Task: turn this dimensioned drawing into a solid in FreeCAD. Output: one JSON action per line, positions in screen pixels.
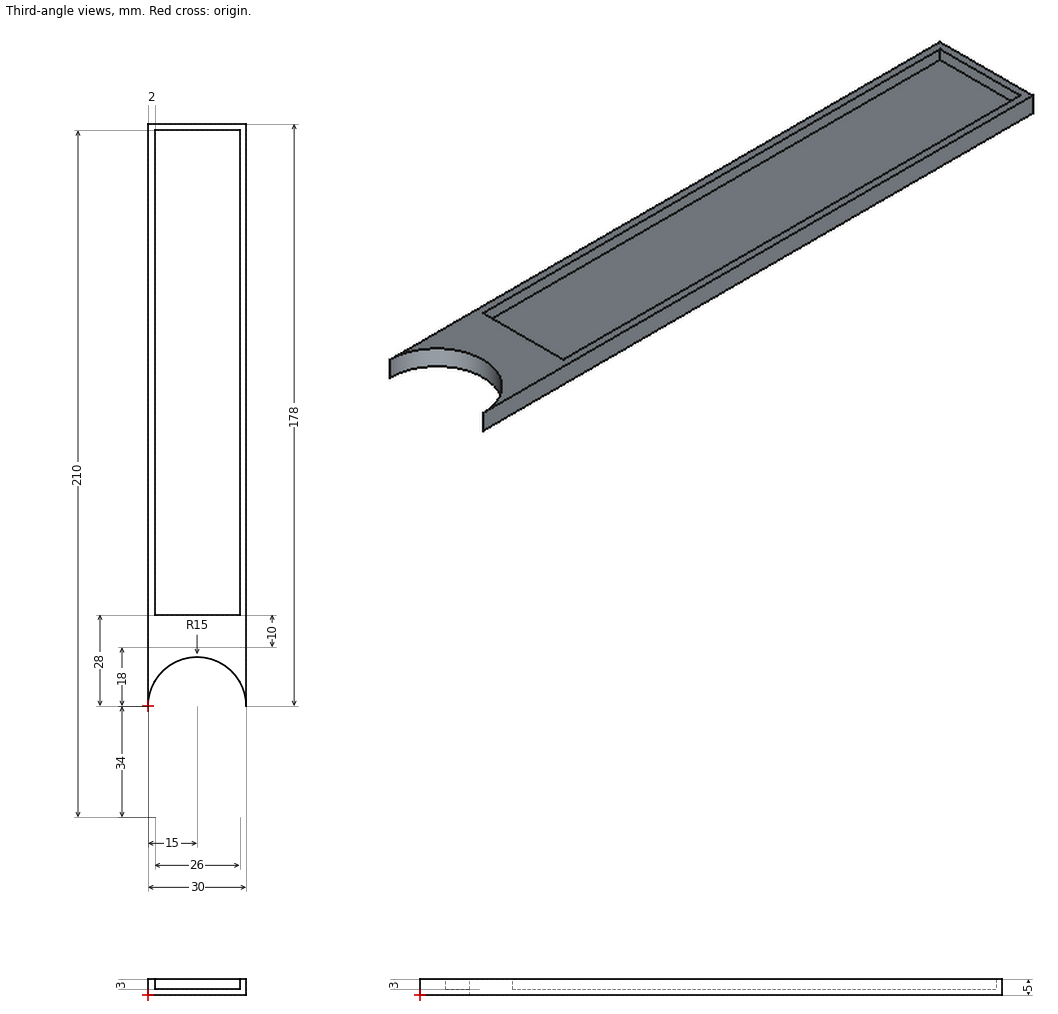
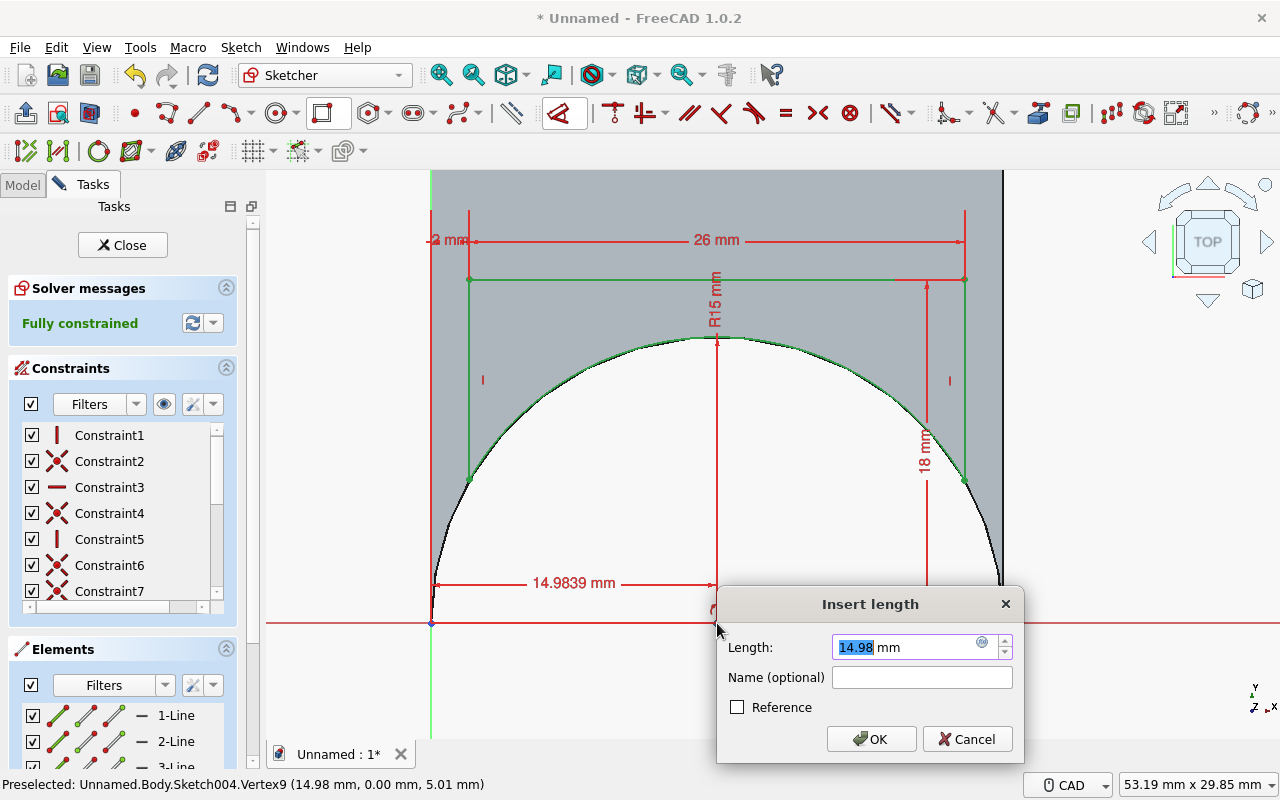
{"action": "type", "text": "15"}
{"action": "key", "text": "Return"}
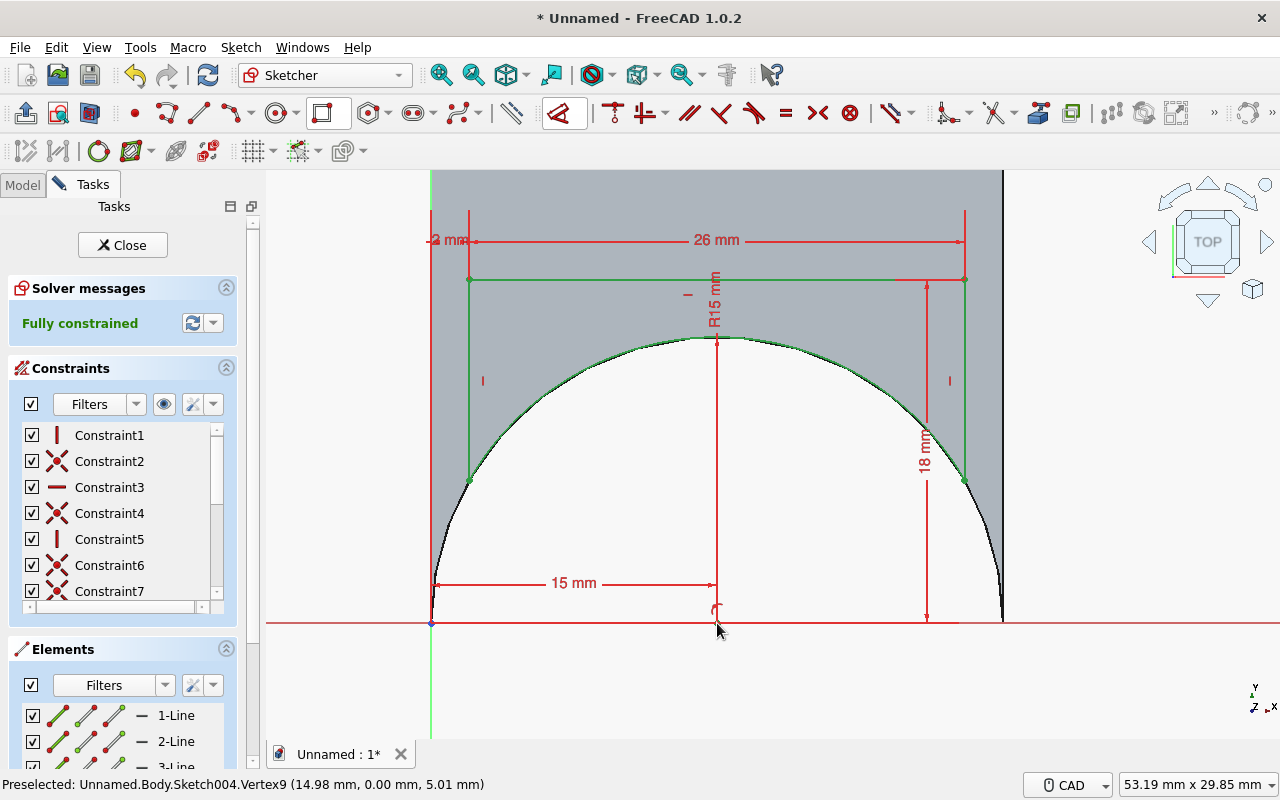
{"action": "left_click", "coordinate": [123, 245]}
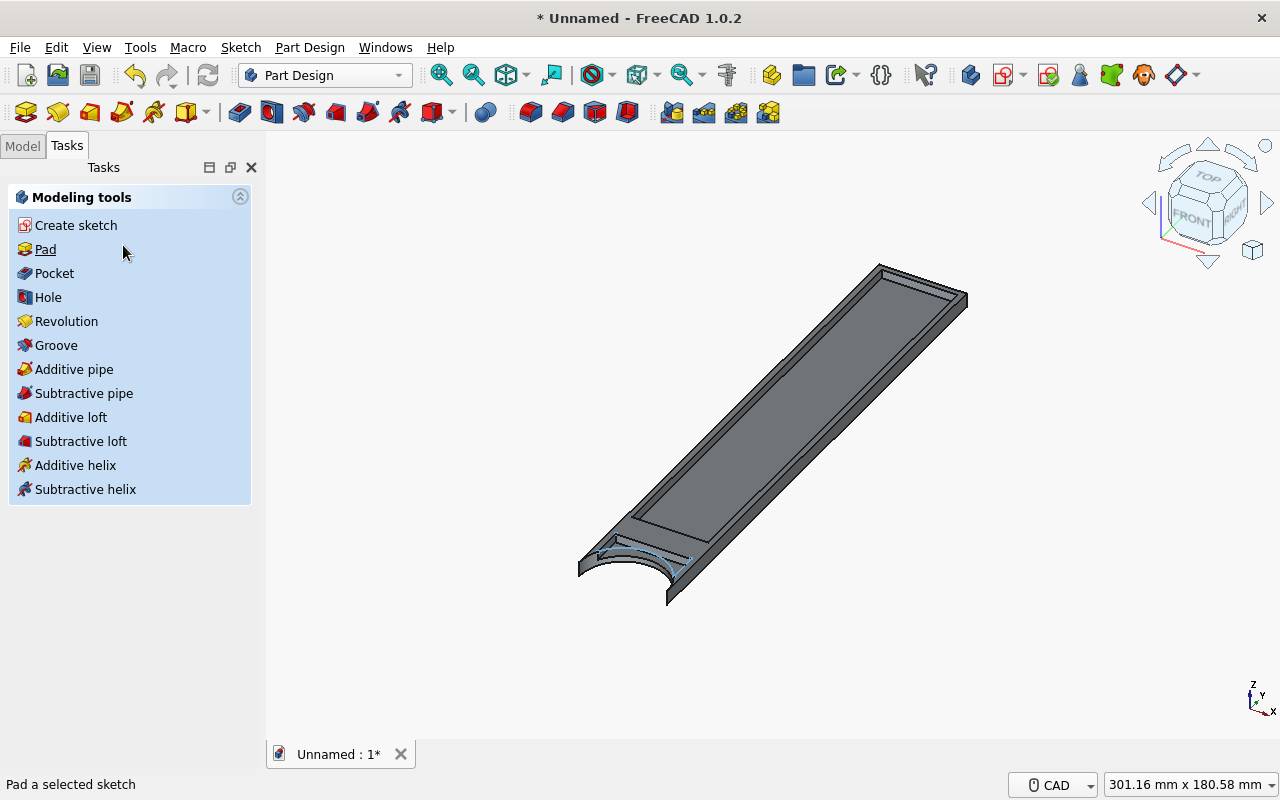
{"action": "left_click", "coordinate": [26, 112]}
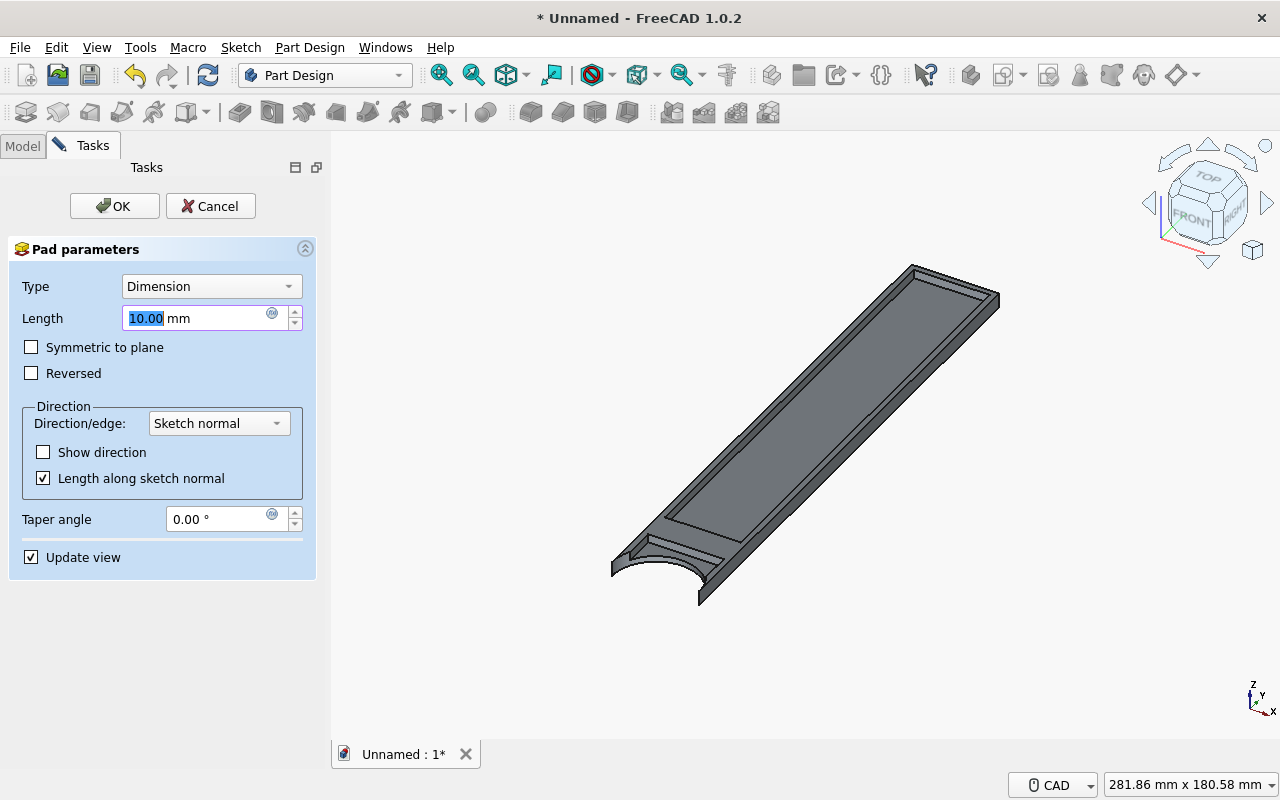
{"action": "type", "text": "3"}
{"action": "key", "text": "Tab"}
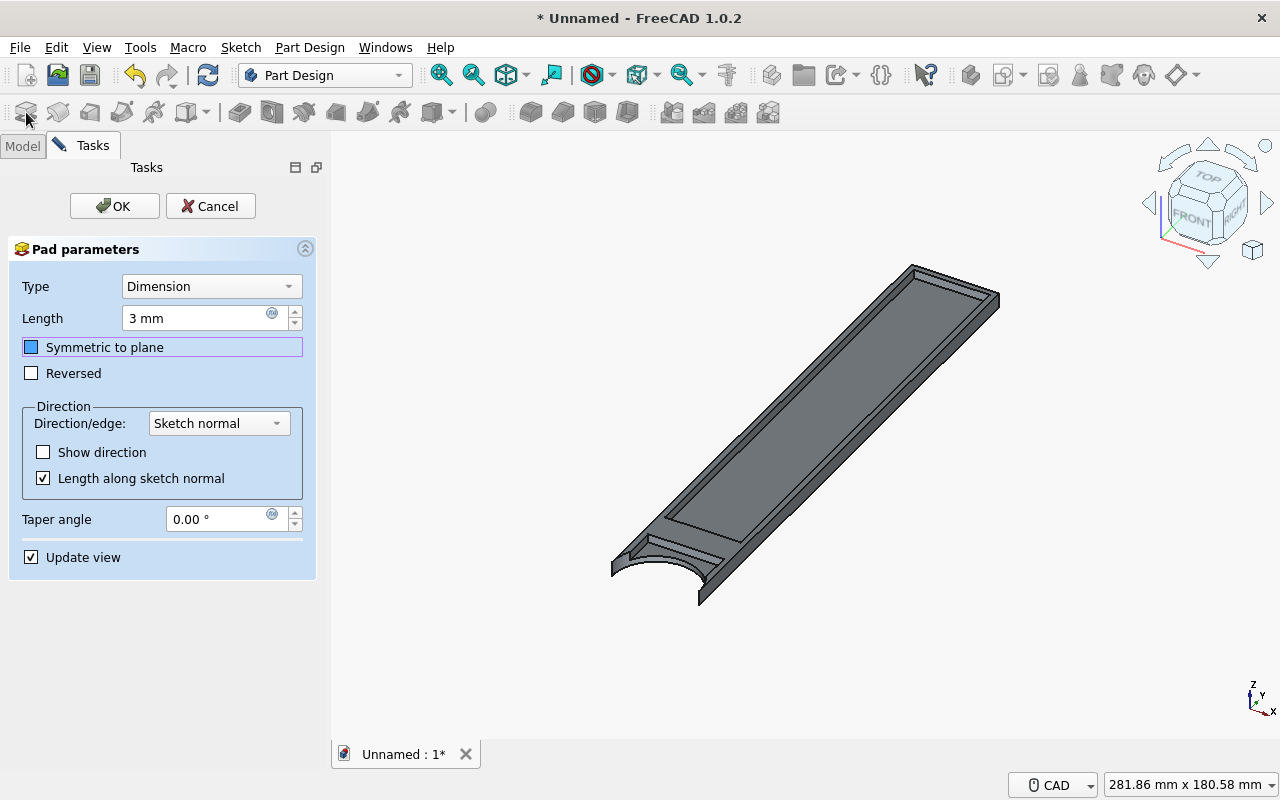
{"action": "left_click", "coordinate": [30, 373]}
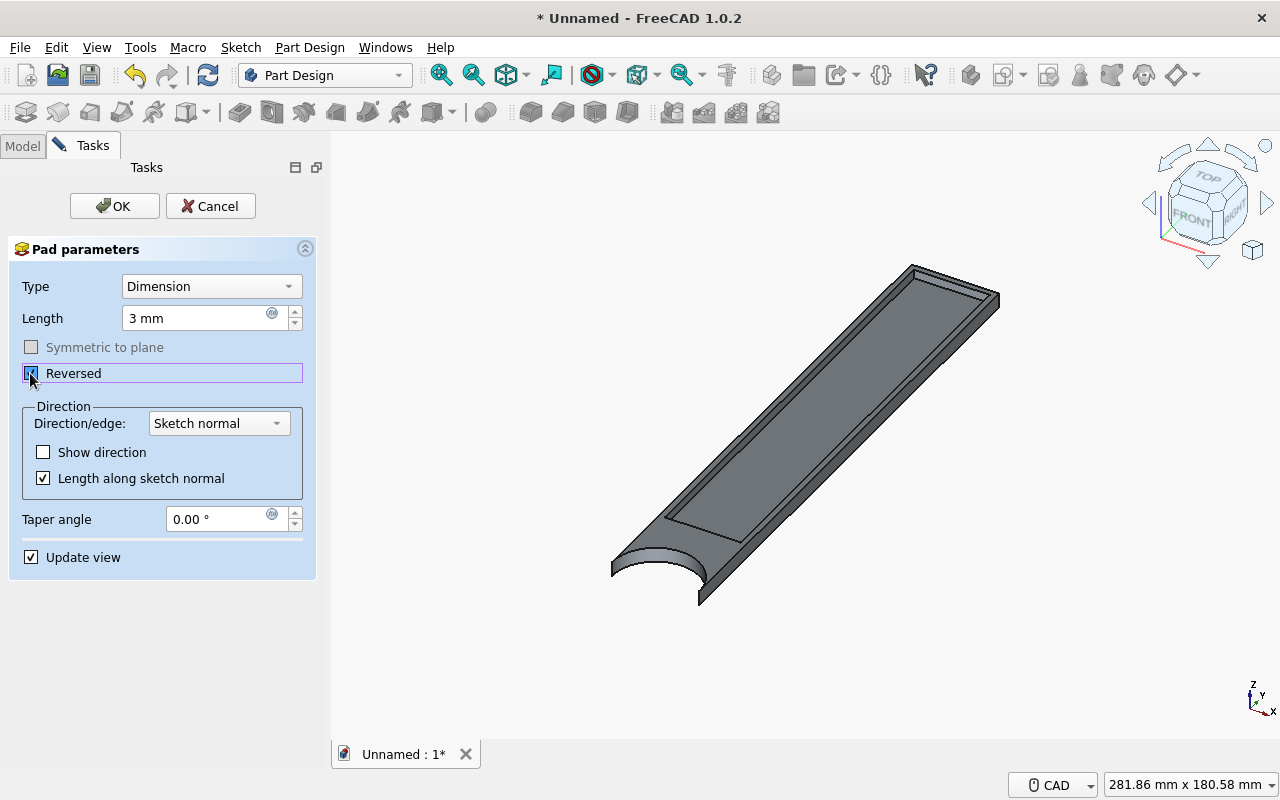
{"action": "left_click", "coordinate": [115, 206]}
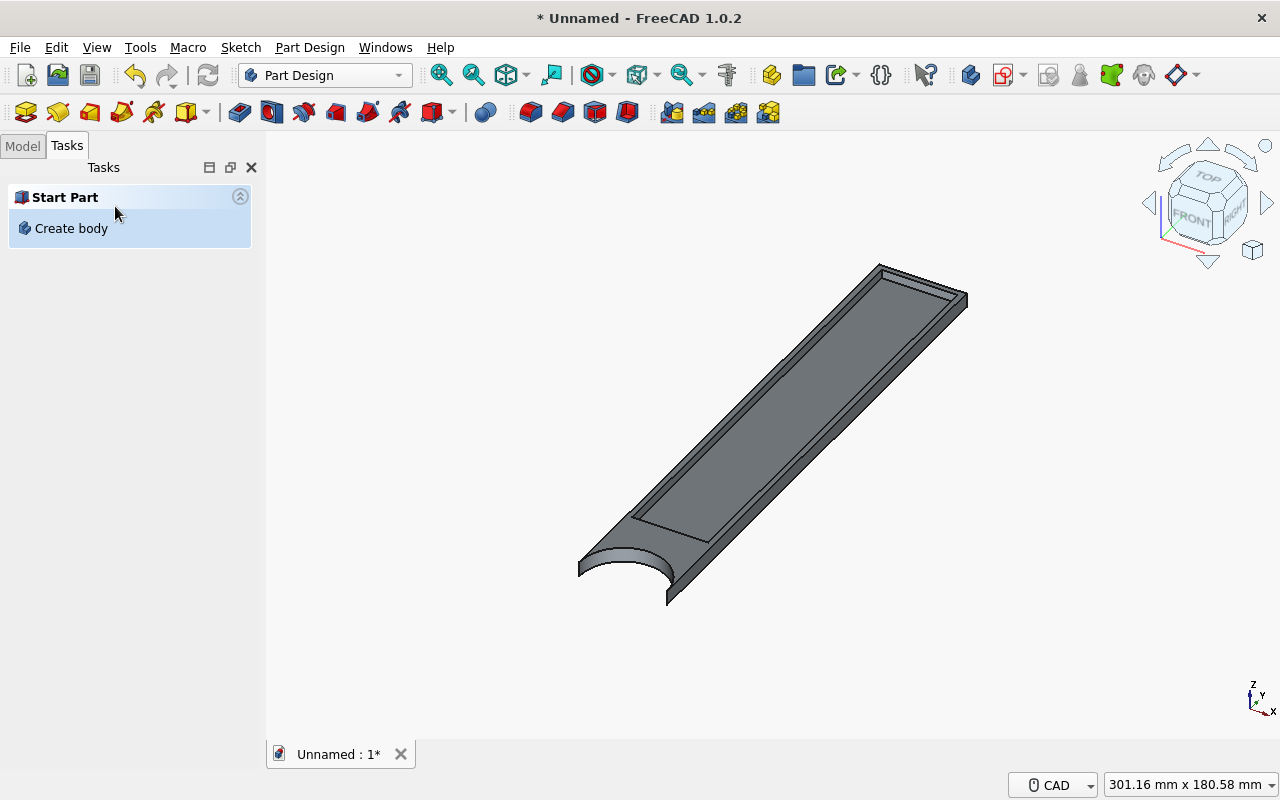
{"action": "key", "text": "0"}